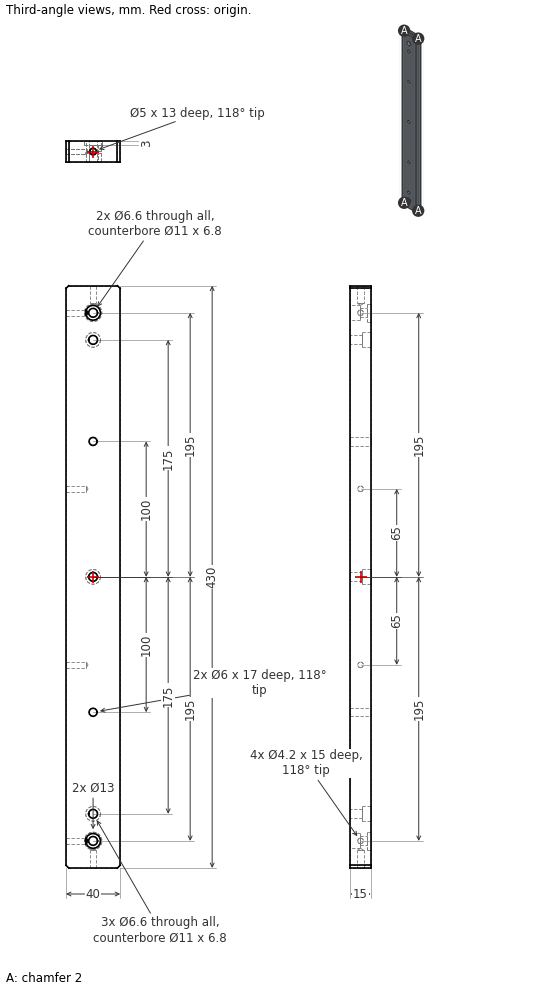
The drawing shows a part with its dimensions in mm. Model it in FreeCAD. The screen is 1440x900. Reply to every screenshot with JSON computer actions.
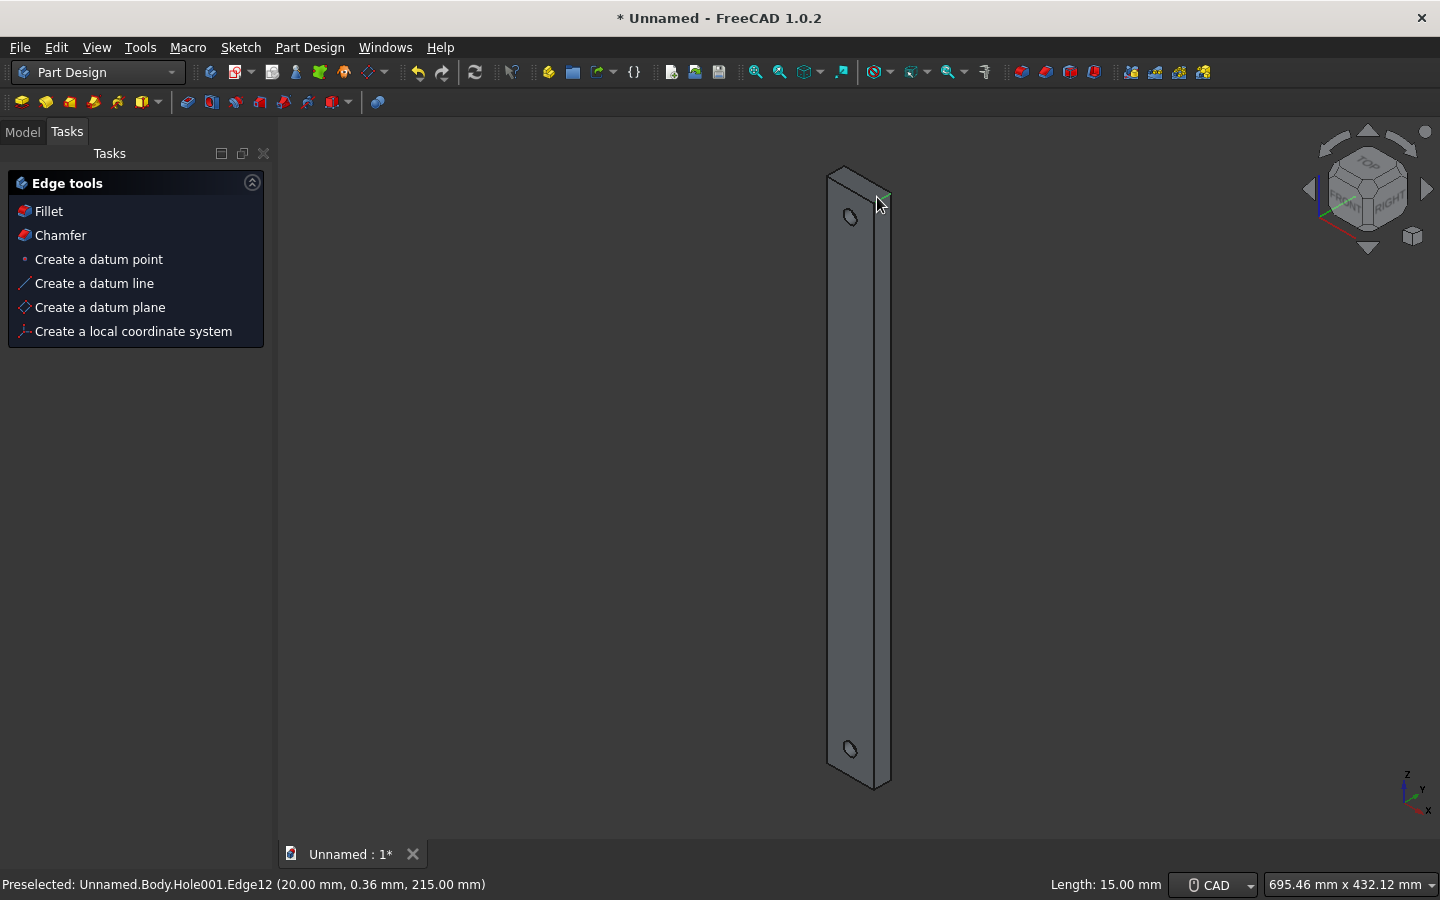
{"action": "key", "text": "2"}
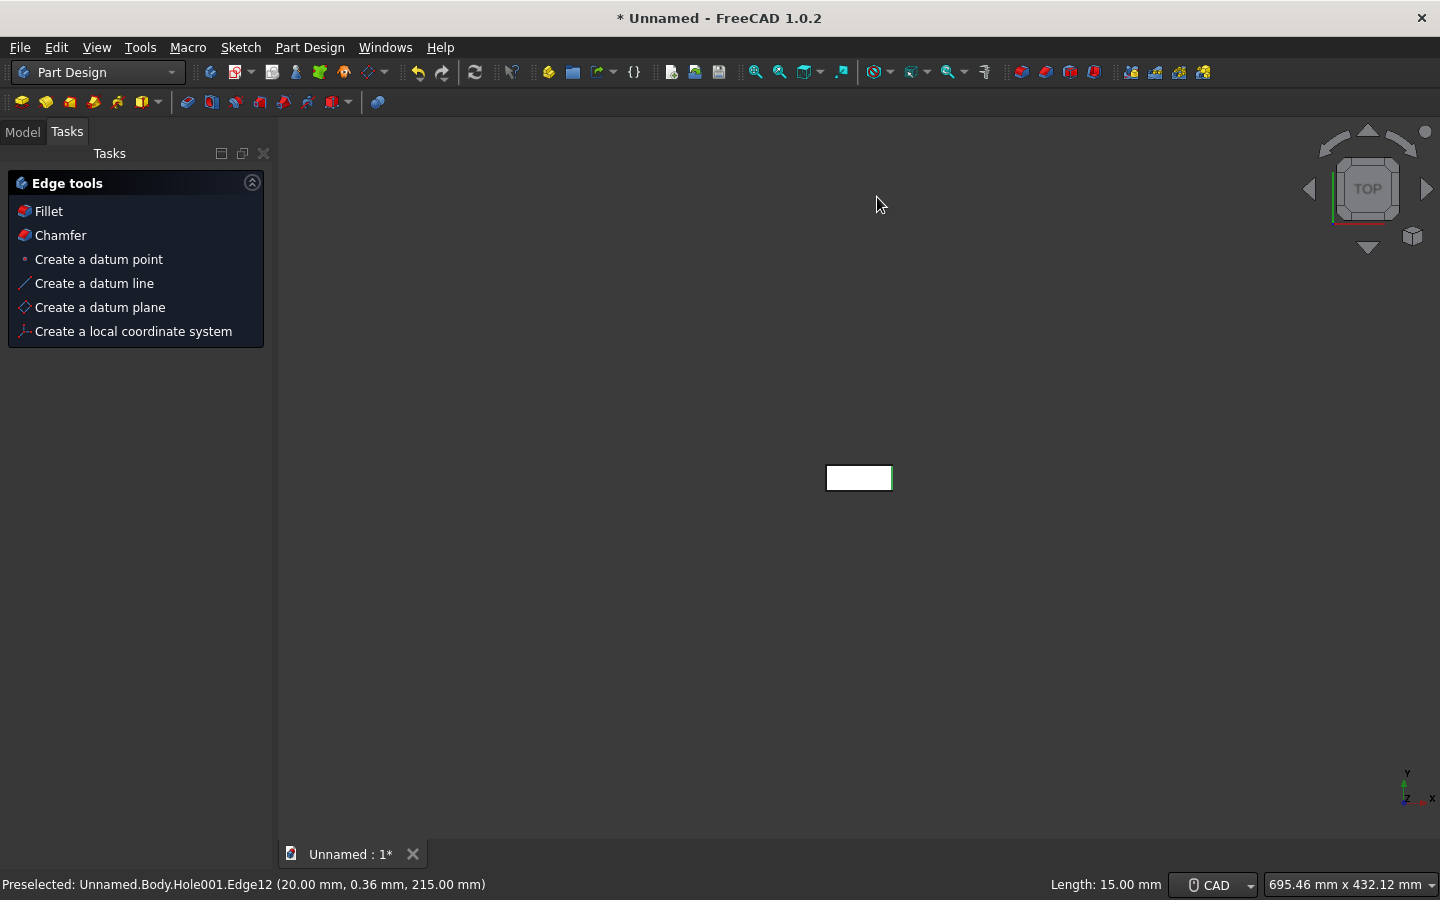
{"action": "key", "text": "v f"}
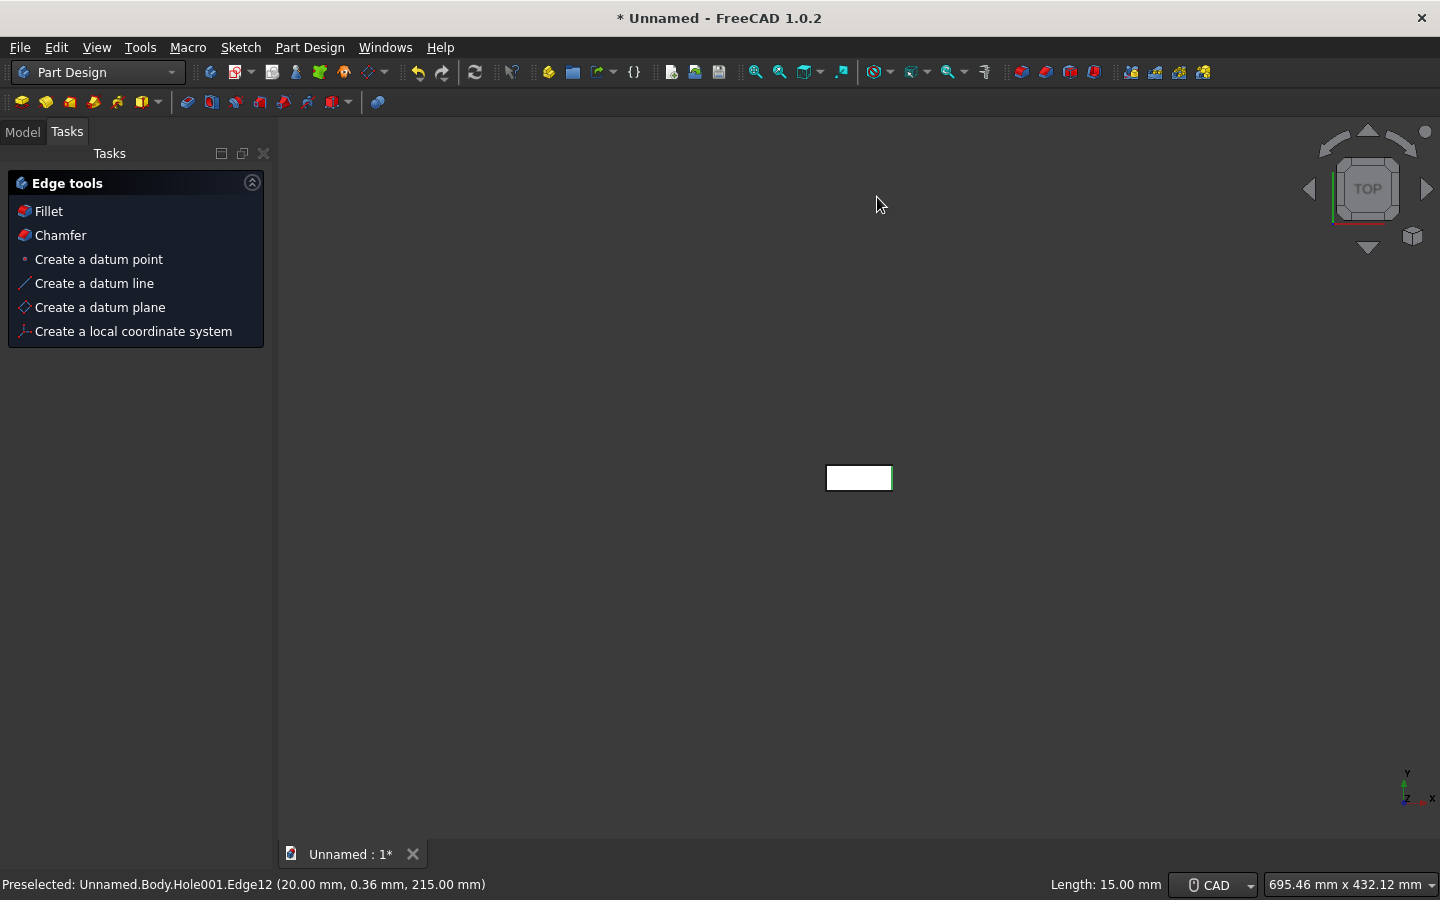
{"action": "left_click", "coordinate": [826, 477], "text": "ctrl"}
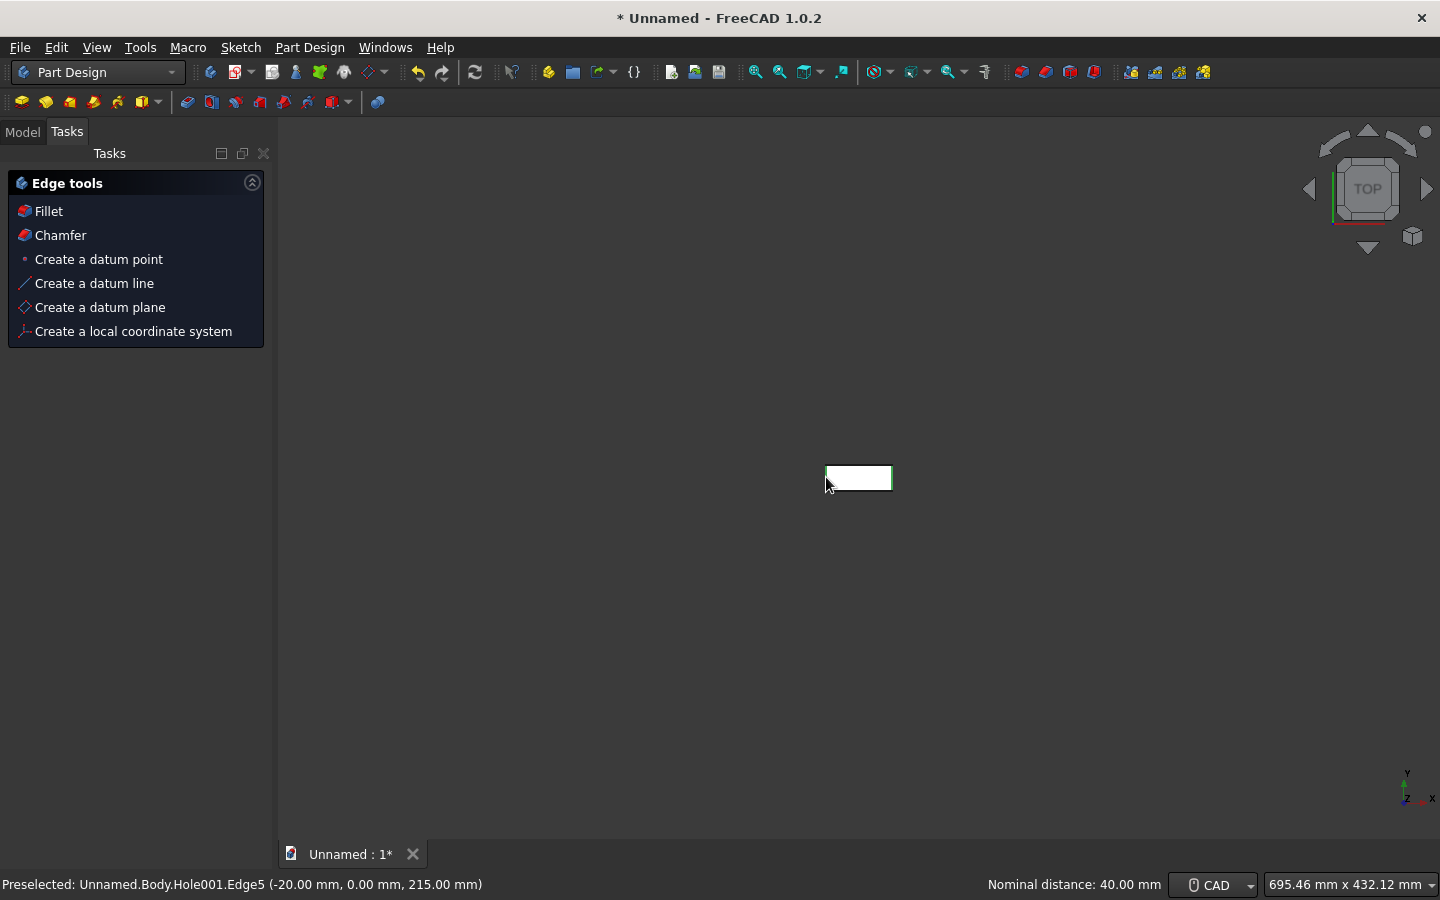
{"action": "key", "text": "1"}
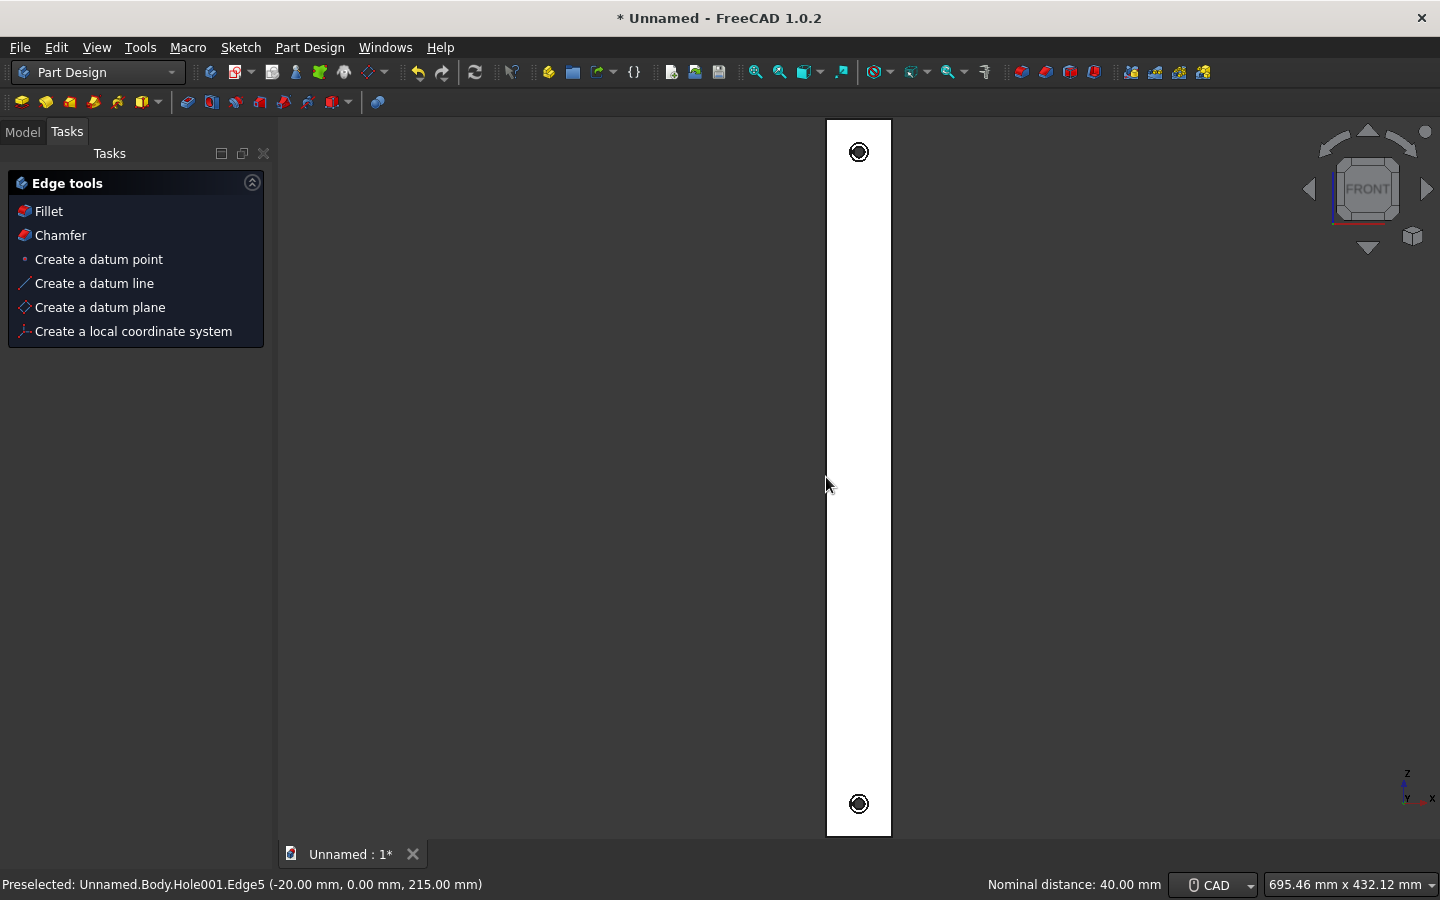
{"action": "key", "text": "3"}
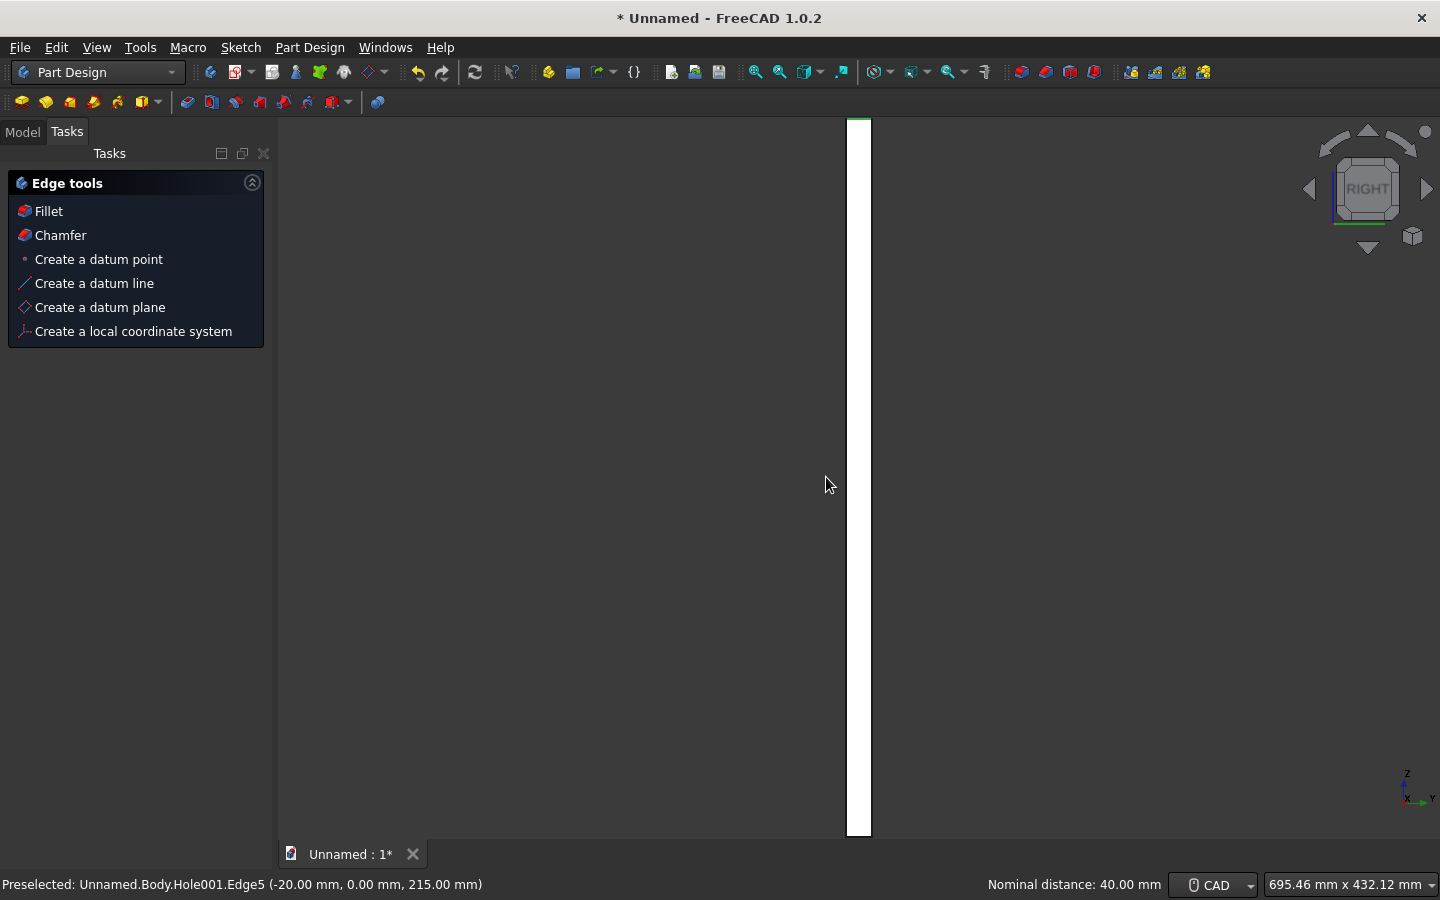
{"action": "key", "text": "5"}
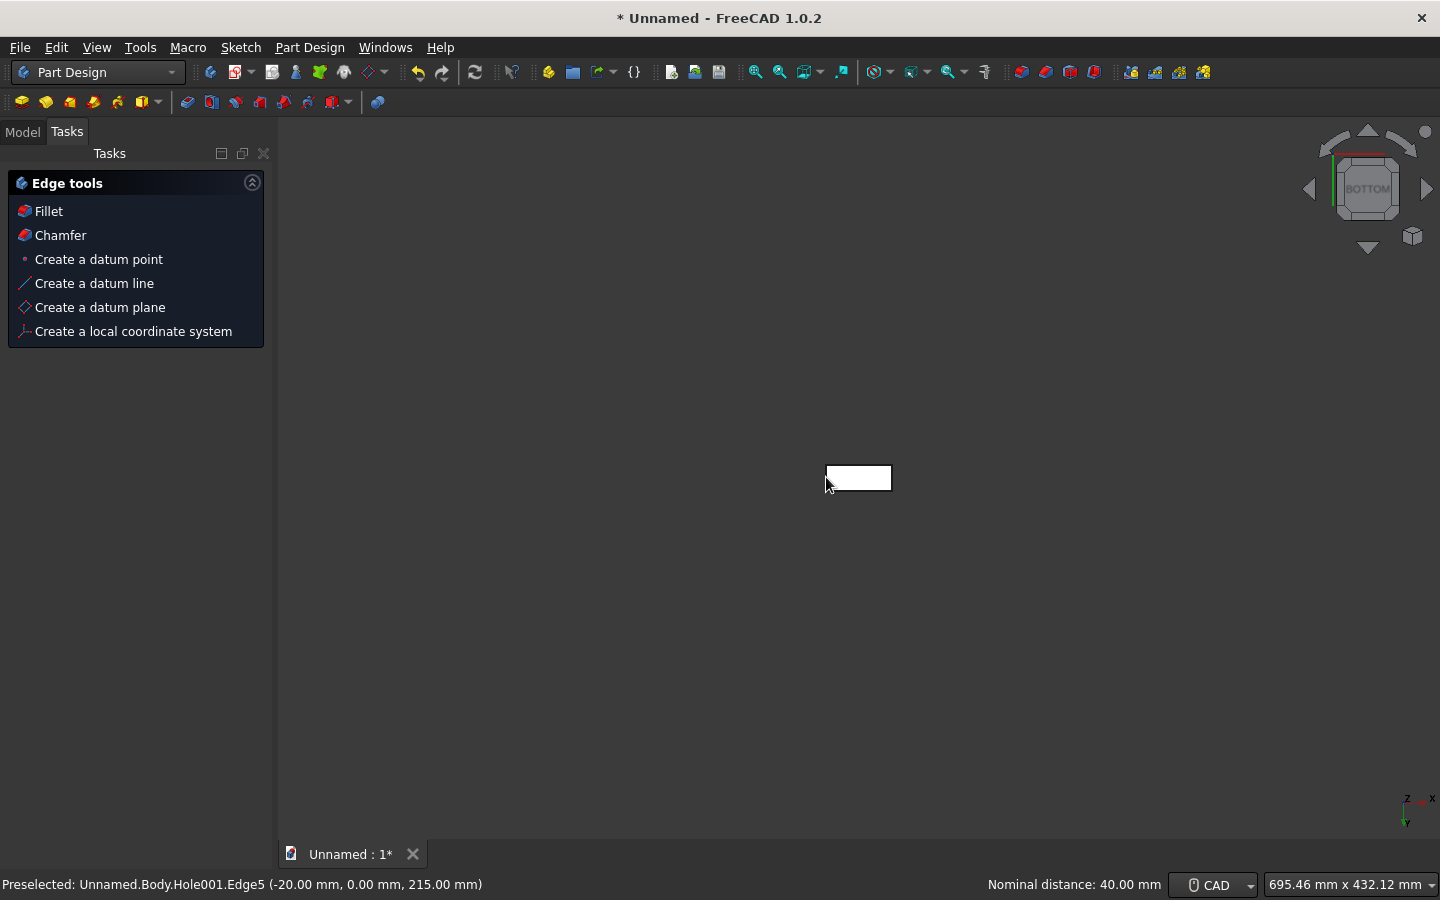
{"action": "key", "text": "v f"}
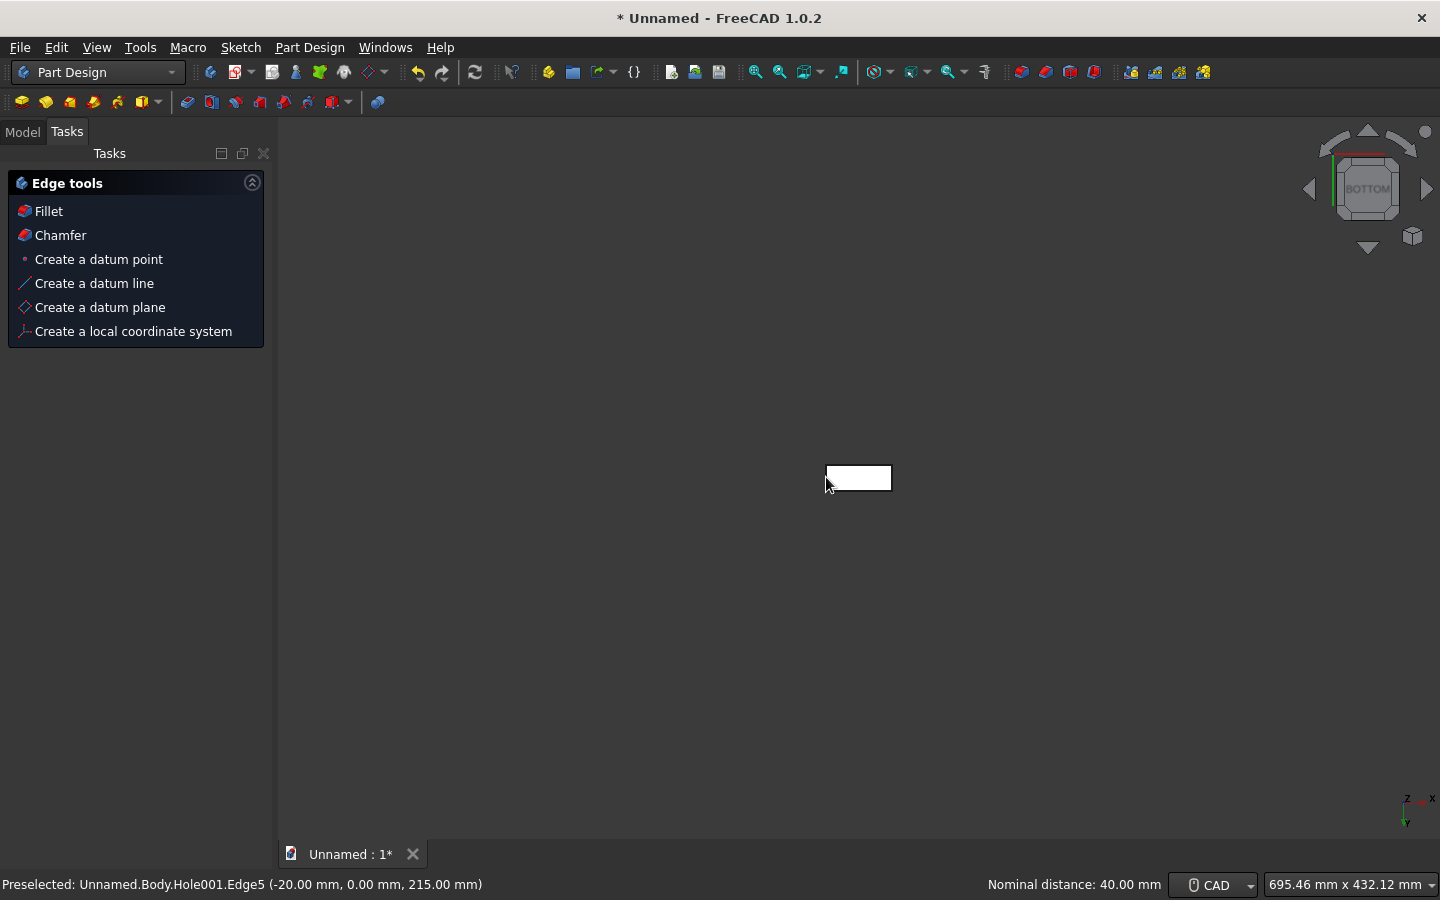
{"action": "left_click", "coordinate": [826, 477], "text": "ctrl"}